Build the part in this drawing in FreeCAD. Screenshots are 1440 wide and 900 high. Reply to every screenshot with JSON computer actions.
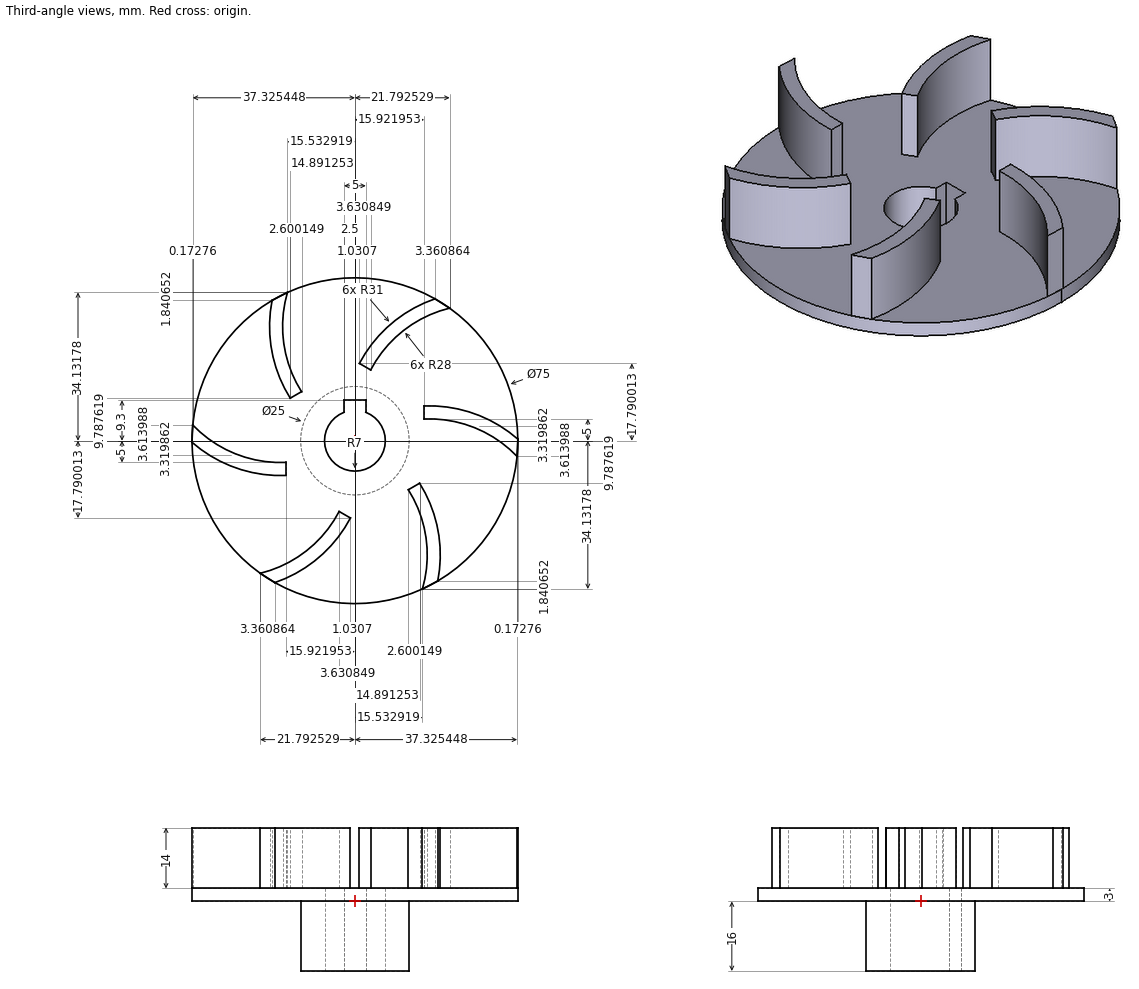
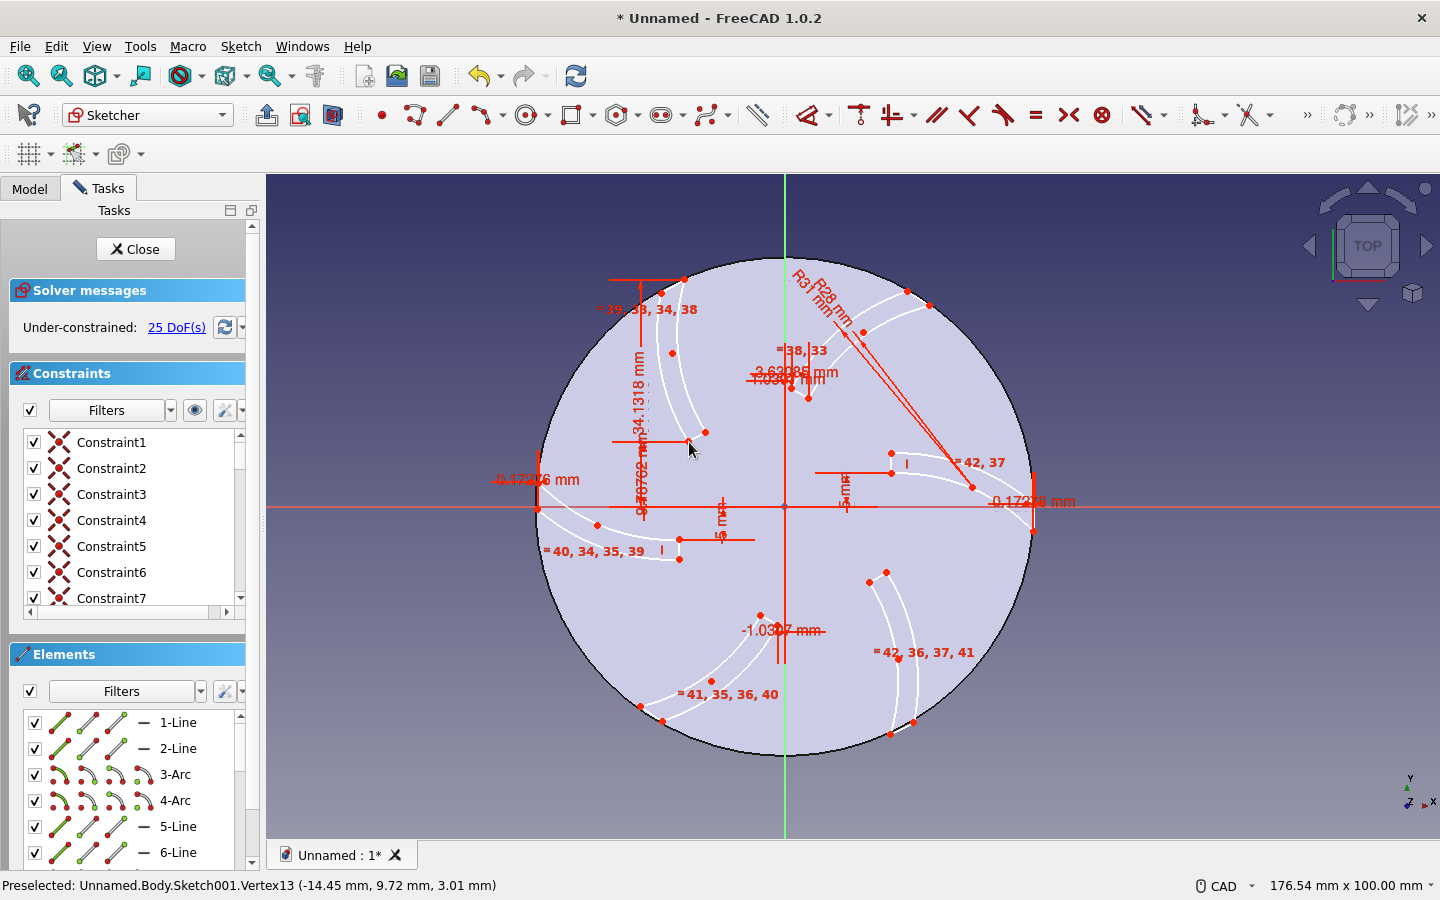
{"action": "scroll", "coordinate": [539, 483], "scroll_direction": "up", "scroll_amount": 3}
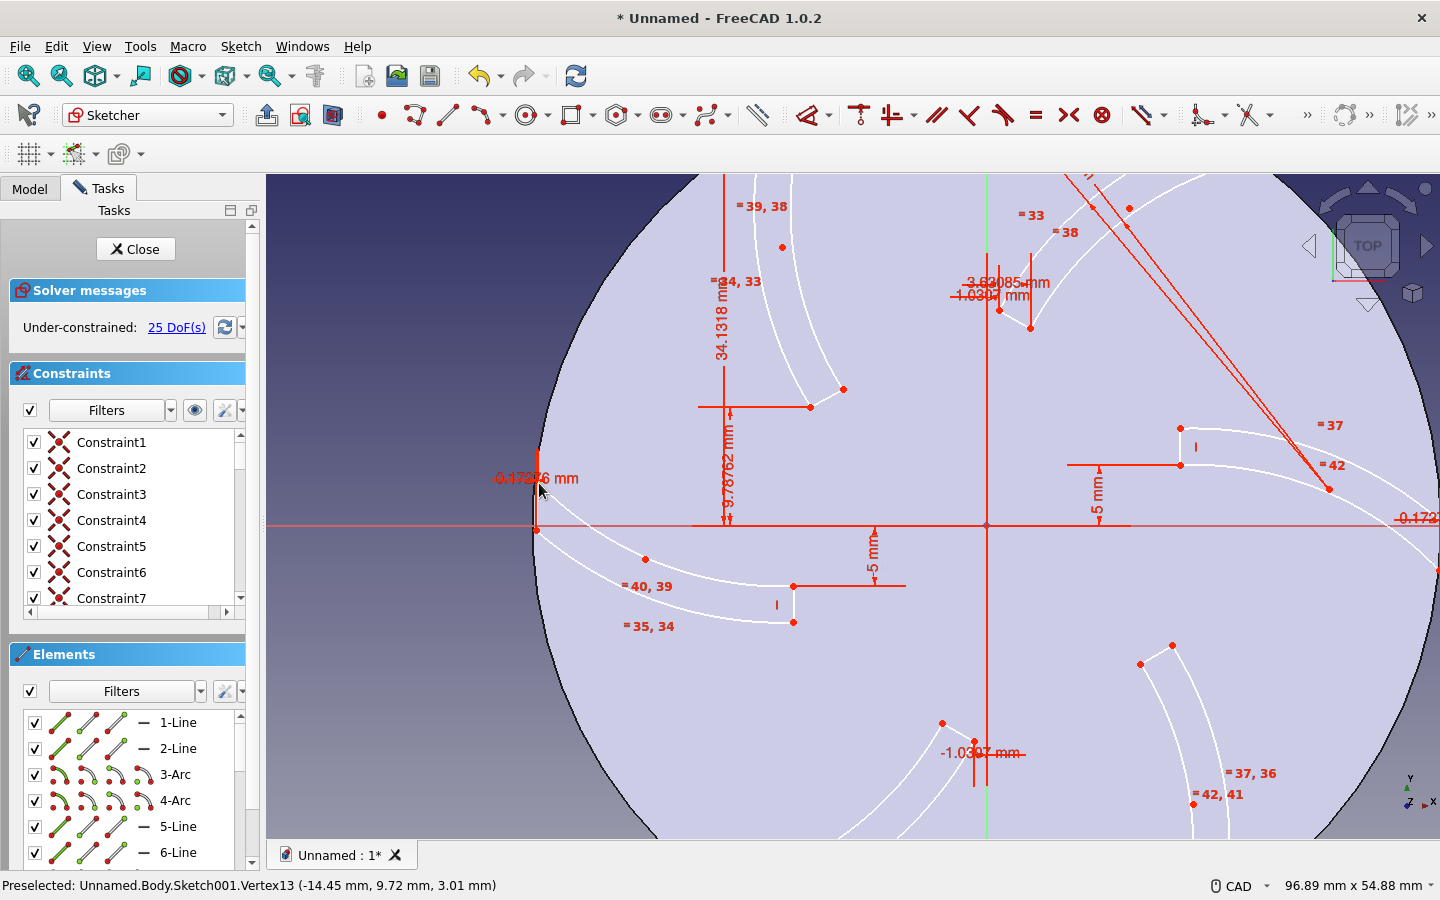
{"action": "left_click", "coordinate": [538, 483]}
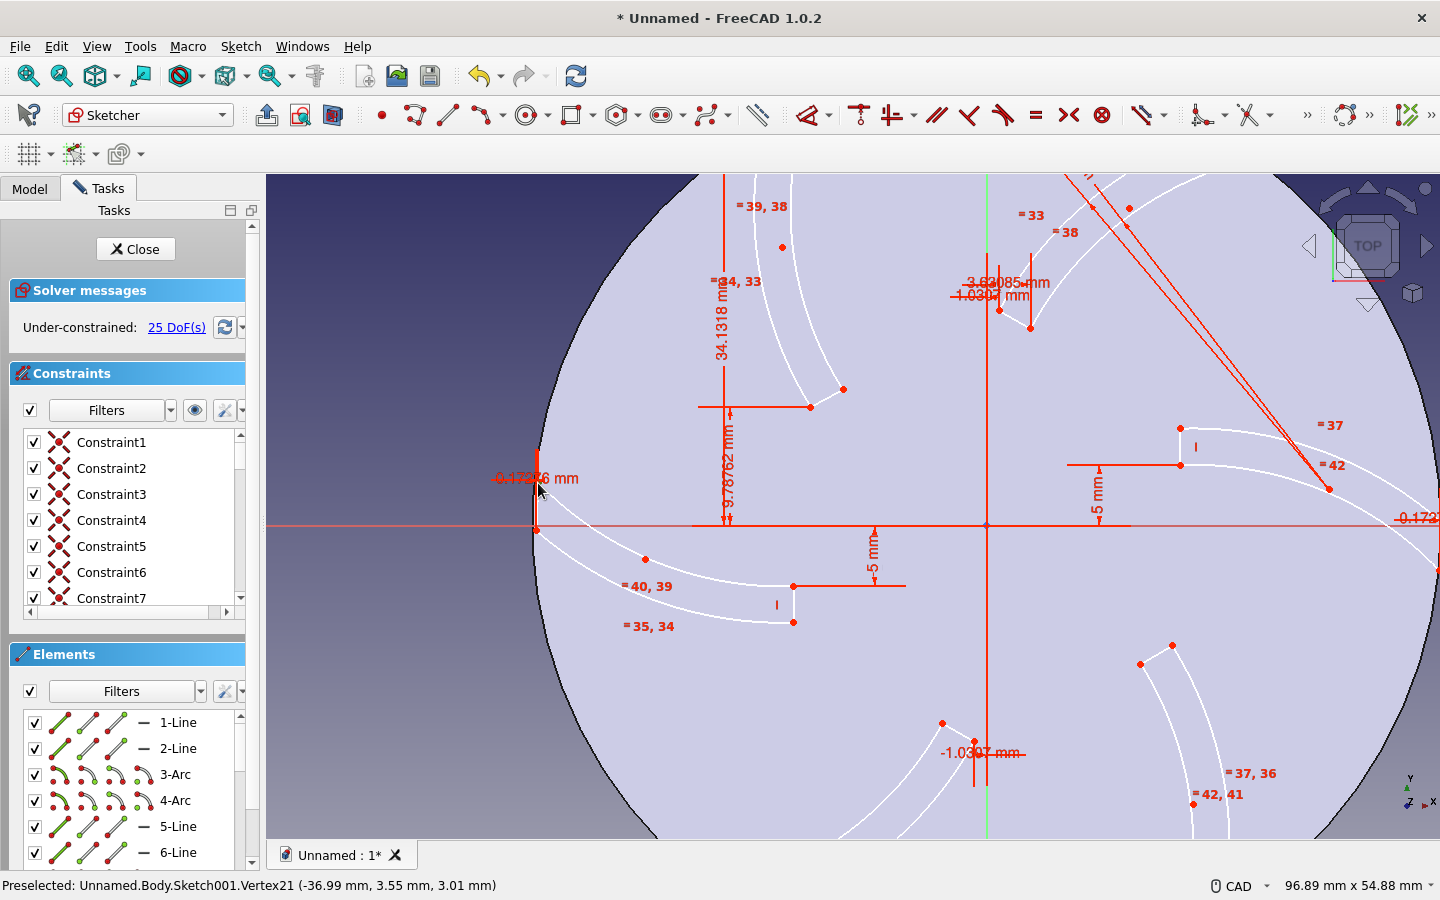
{"action": "left_click", "coordinate": [828, 116]}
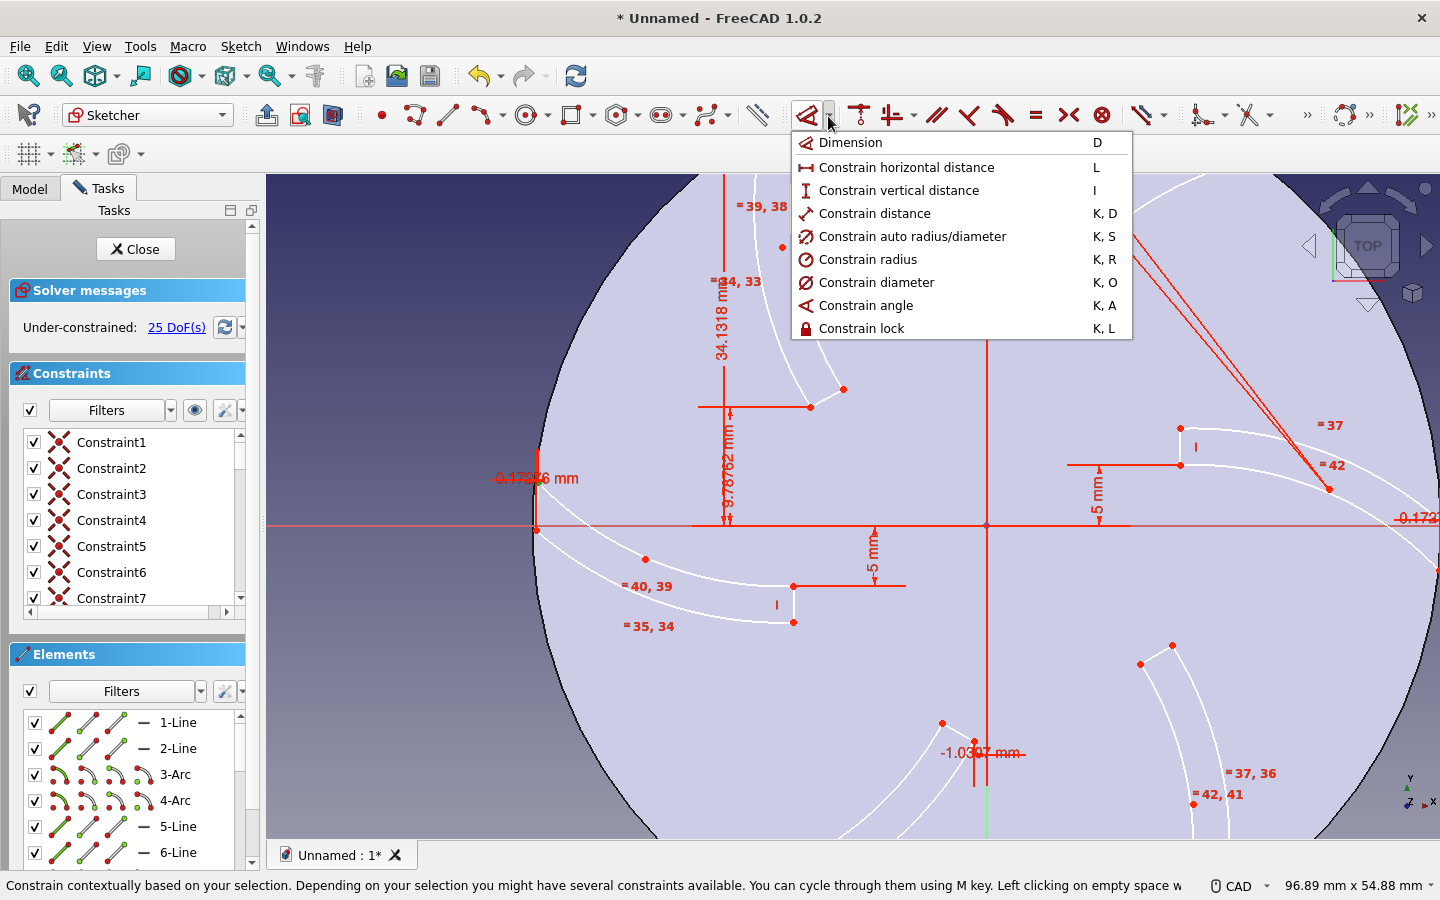
{"action": "left_click", "coordinate": [962, 190]}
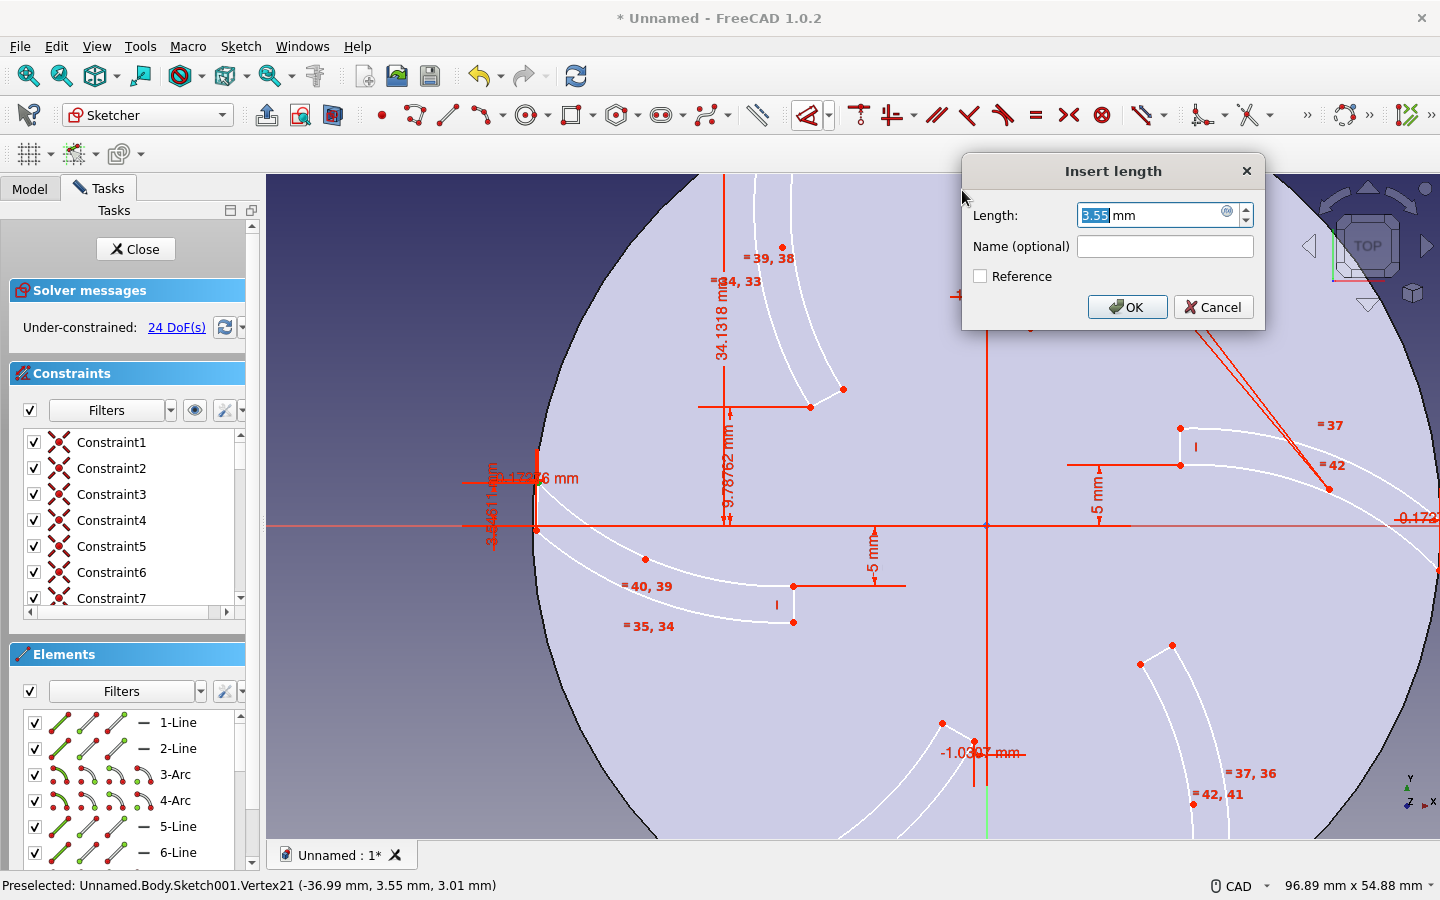
{"action": "type", "text": "3.613988"}
{"action": "key", "text": "Return"}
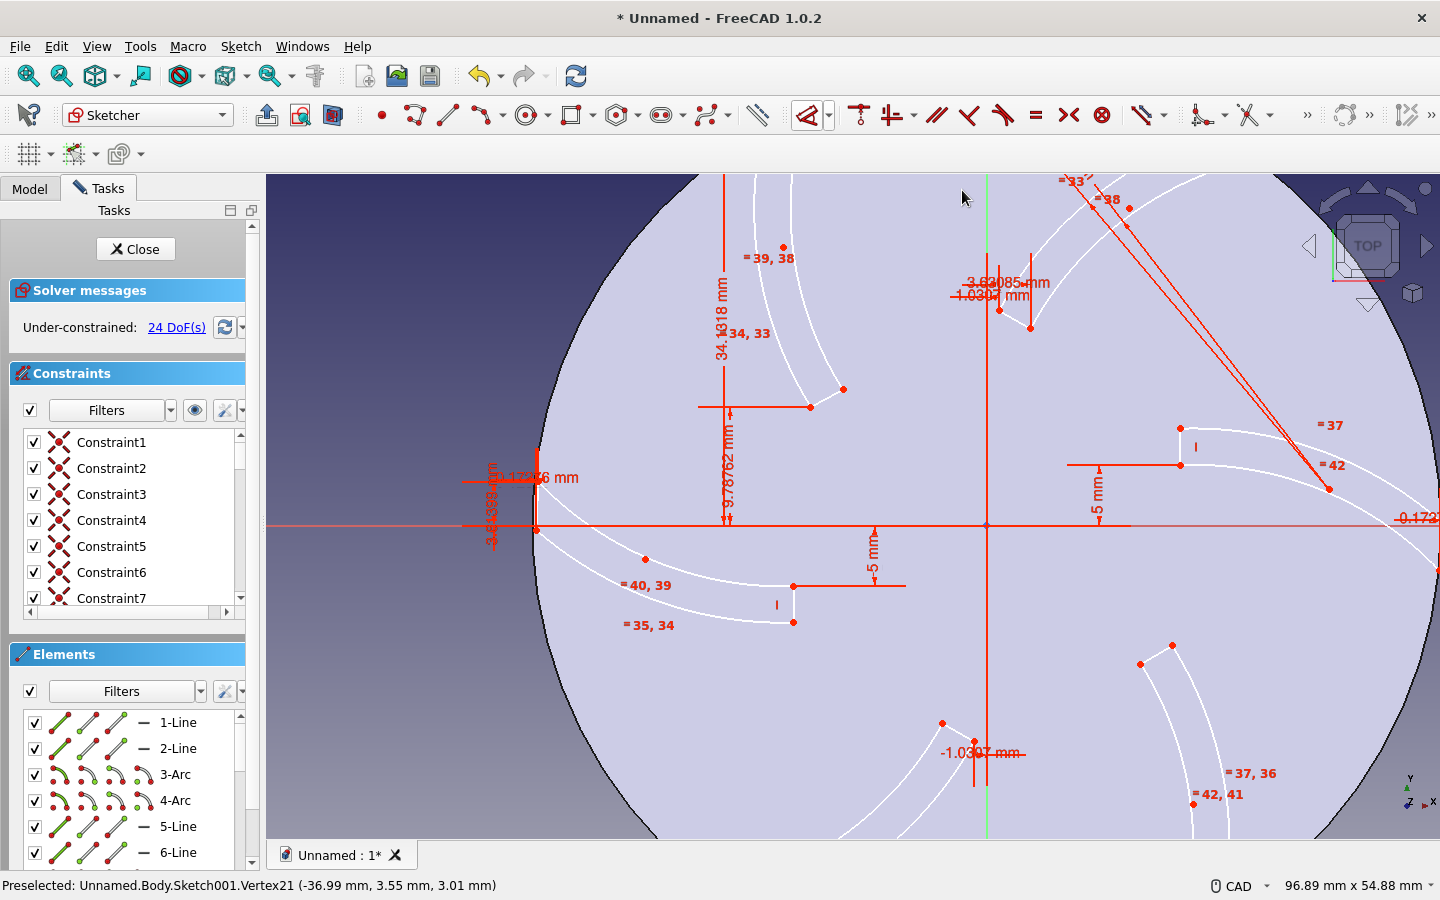
{"action": "left_click", "coordinate": [943, 723]}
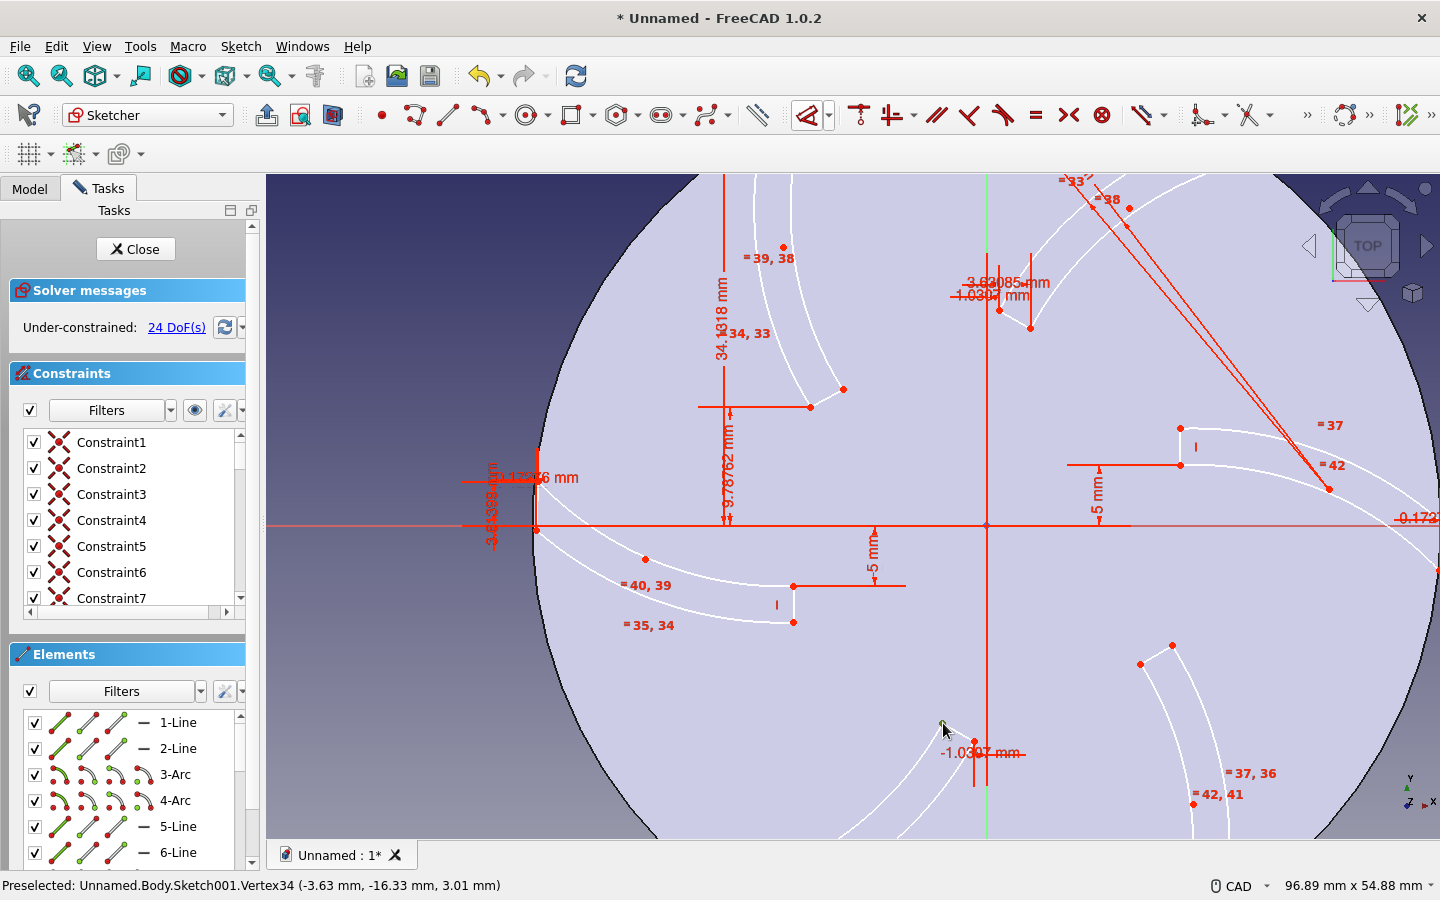
{"action": "key", "text": "l"}